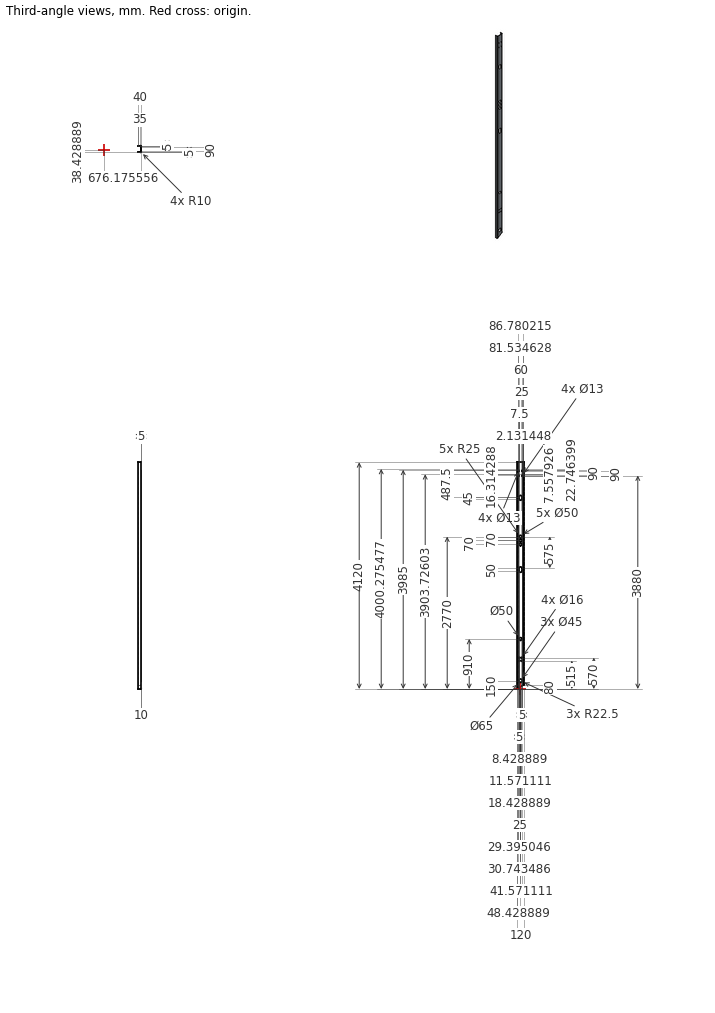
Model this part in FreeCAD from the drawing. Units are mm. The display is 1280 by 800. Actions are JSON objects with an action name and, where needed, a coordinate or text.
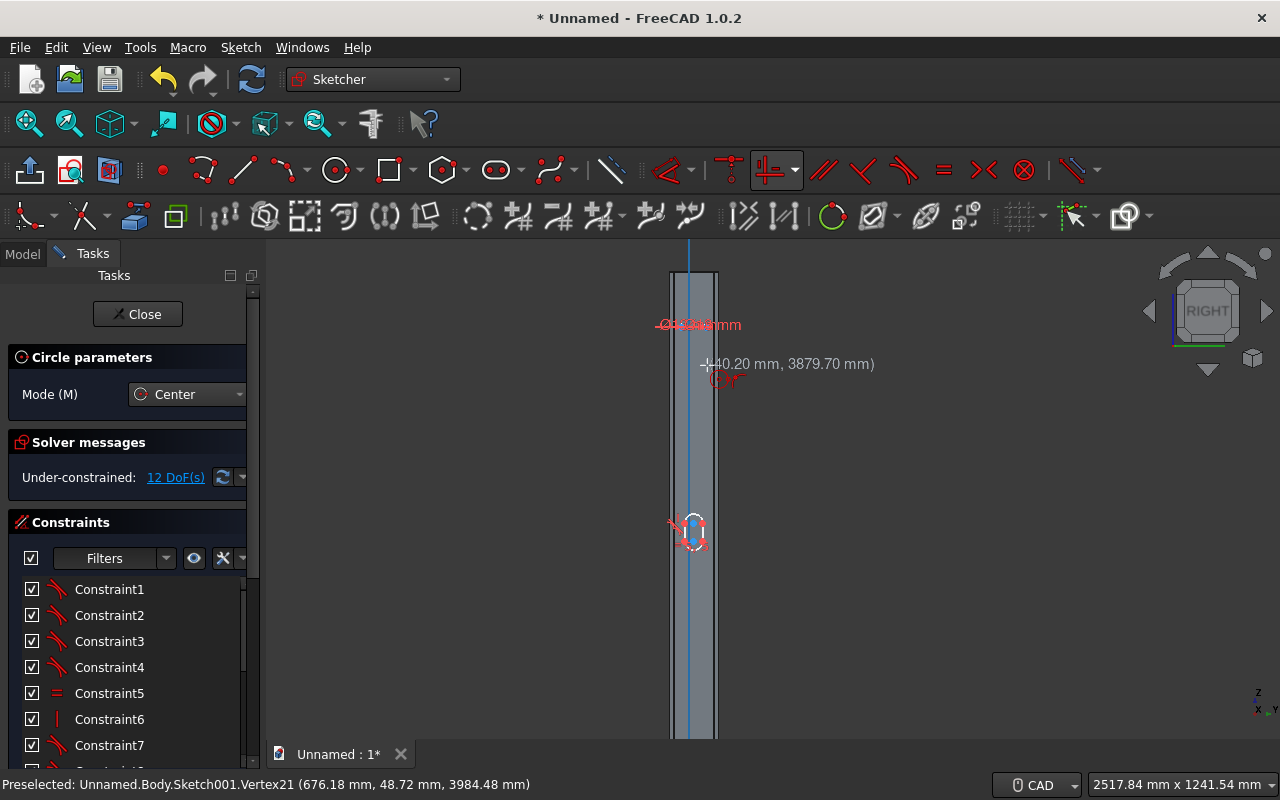
{"action": "left_click", "coordinate": [706, 363]}
{"action": "mouse_move", "coordinate": [708, 361]}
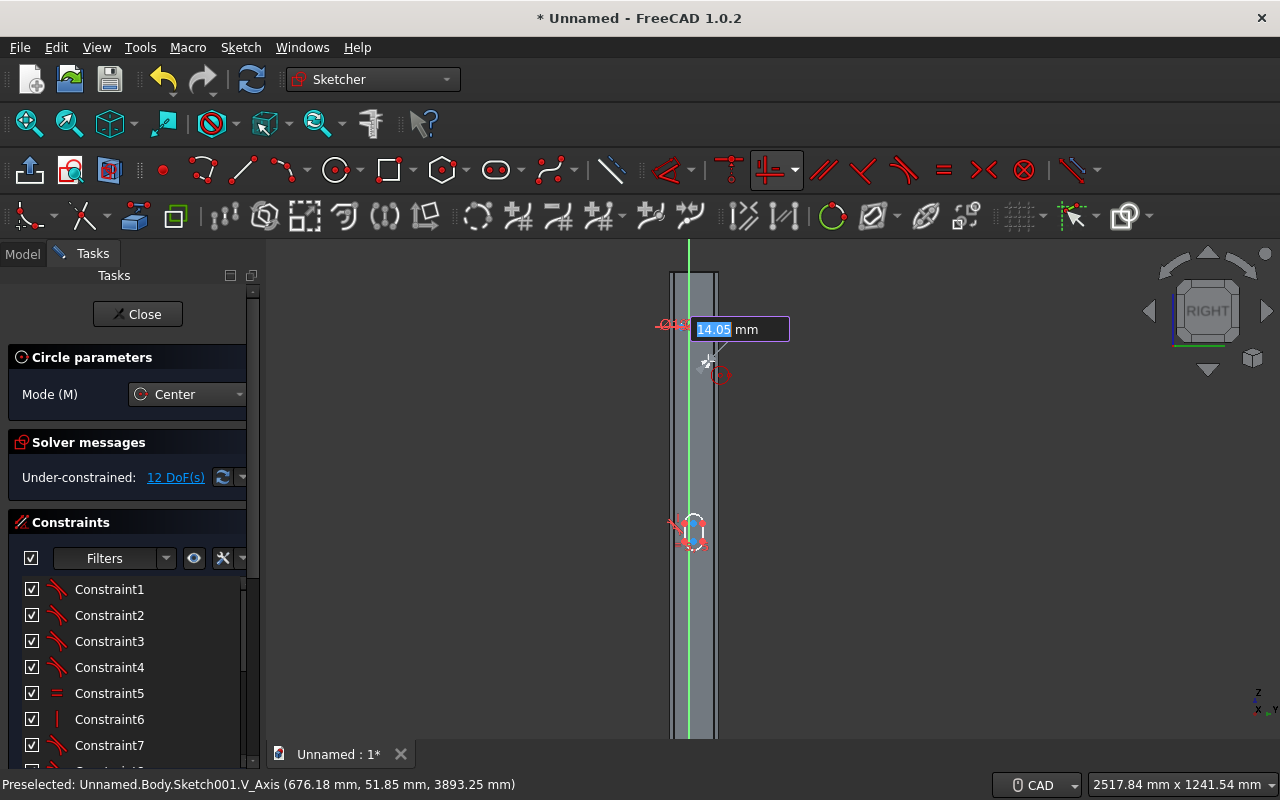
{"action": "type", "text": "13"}
{"action": "key", "text": "Return"}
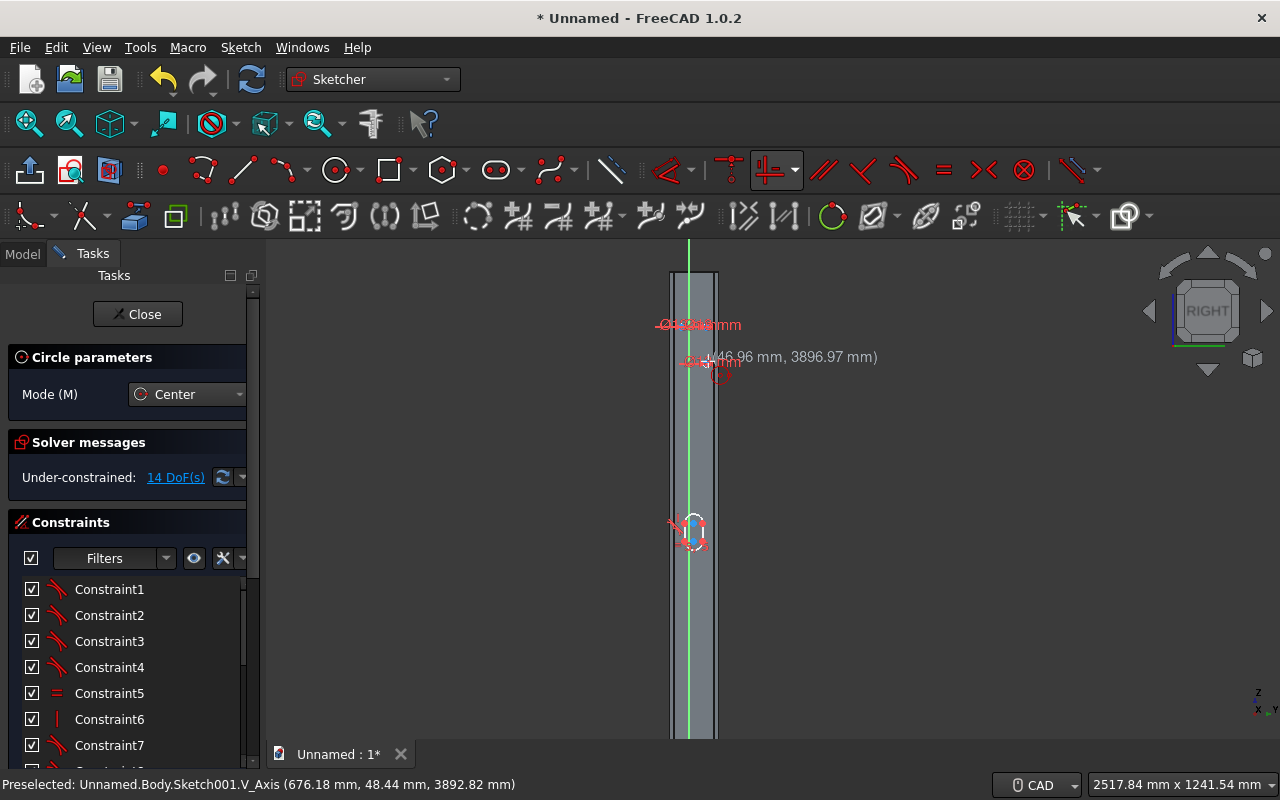
{"action": "scroll", "coordinate": [682, 363], "scroll_direction": "up", "scroll_amount": 11}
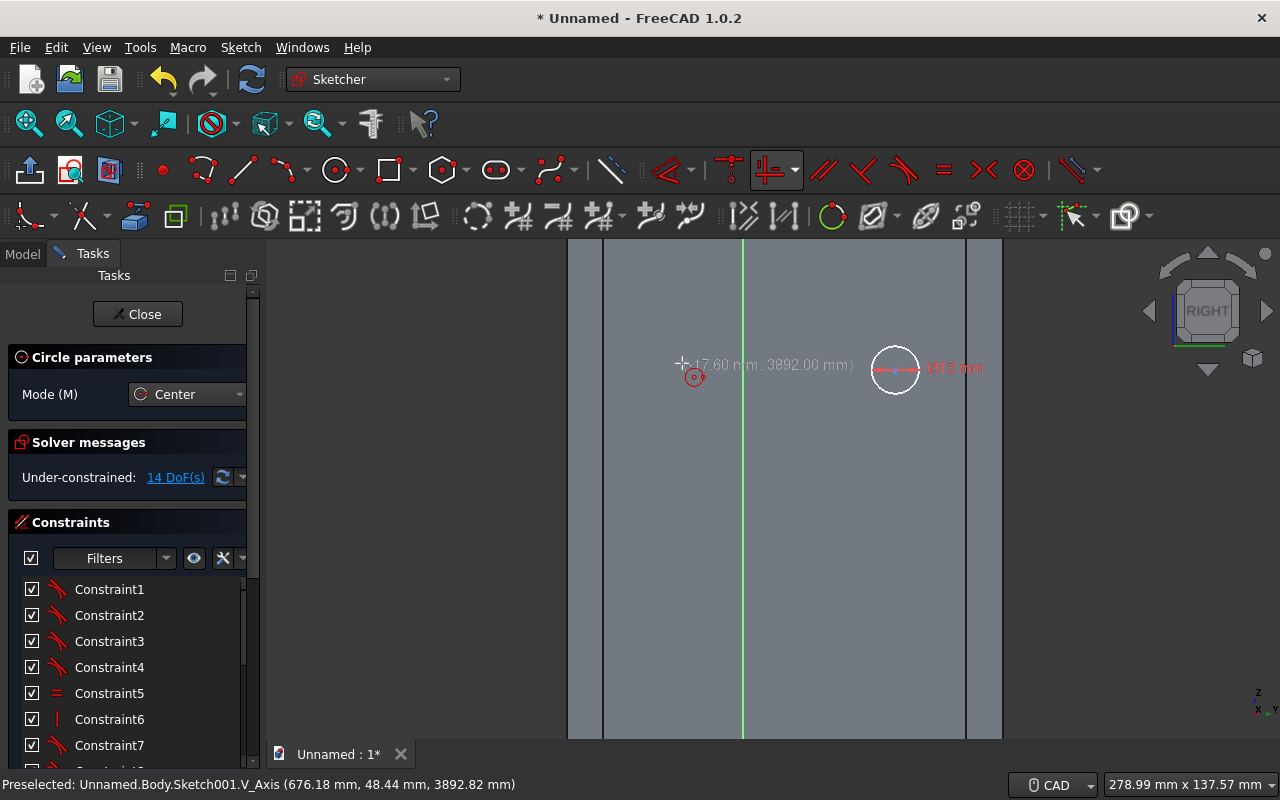
{"action": "scroll", "coordinate": [704, 489], "scroll_direction": "down", "scroll_amount": 15}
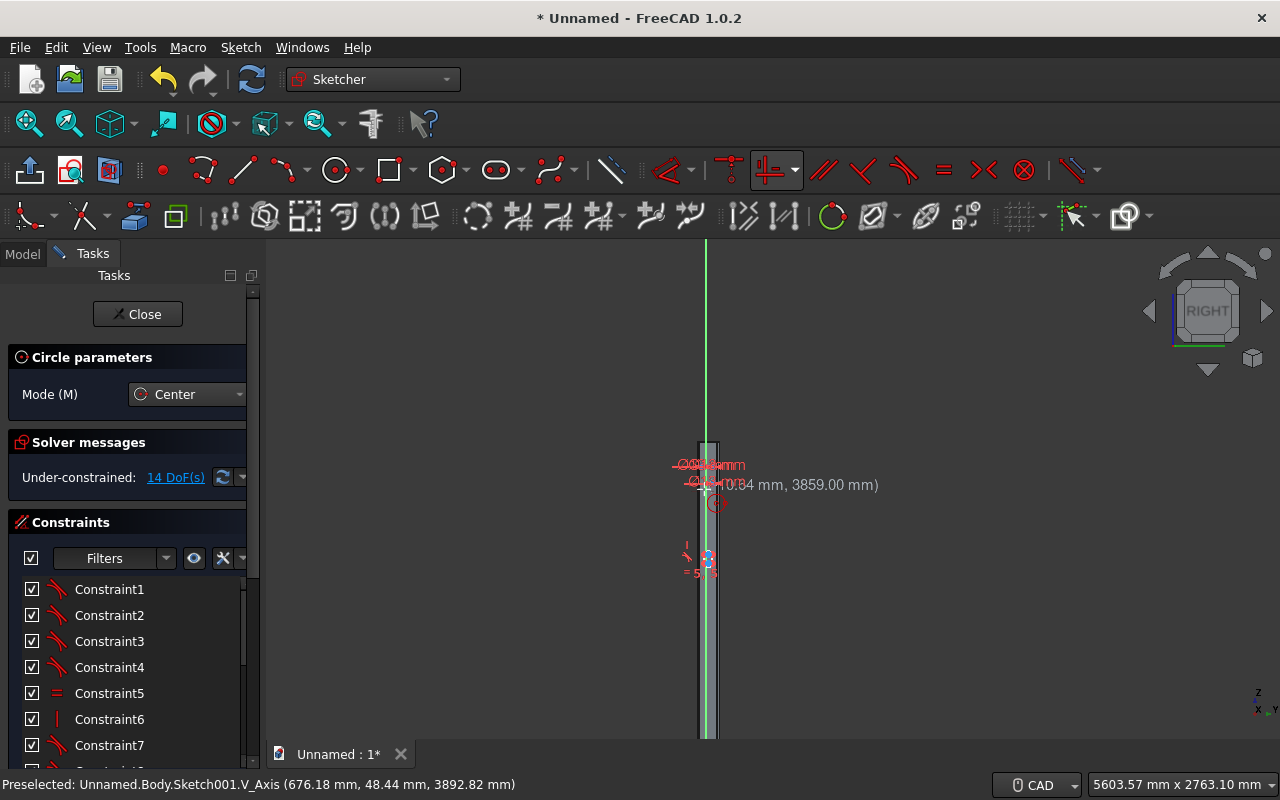
{"action": "scroll", "coordinate": [701, 267], "scroll_direction": "down", "scroll_amount": 4}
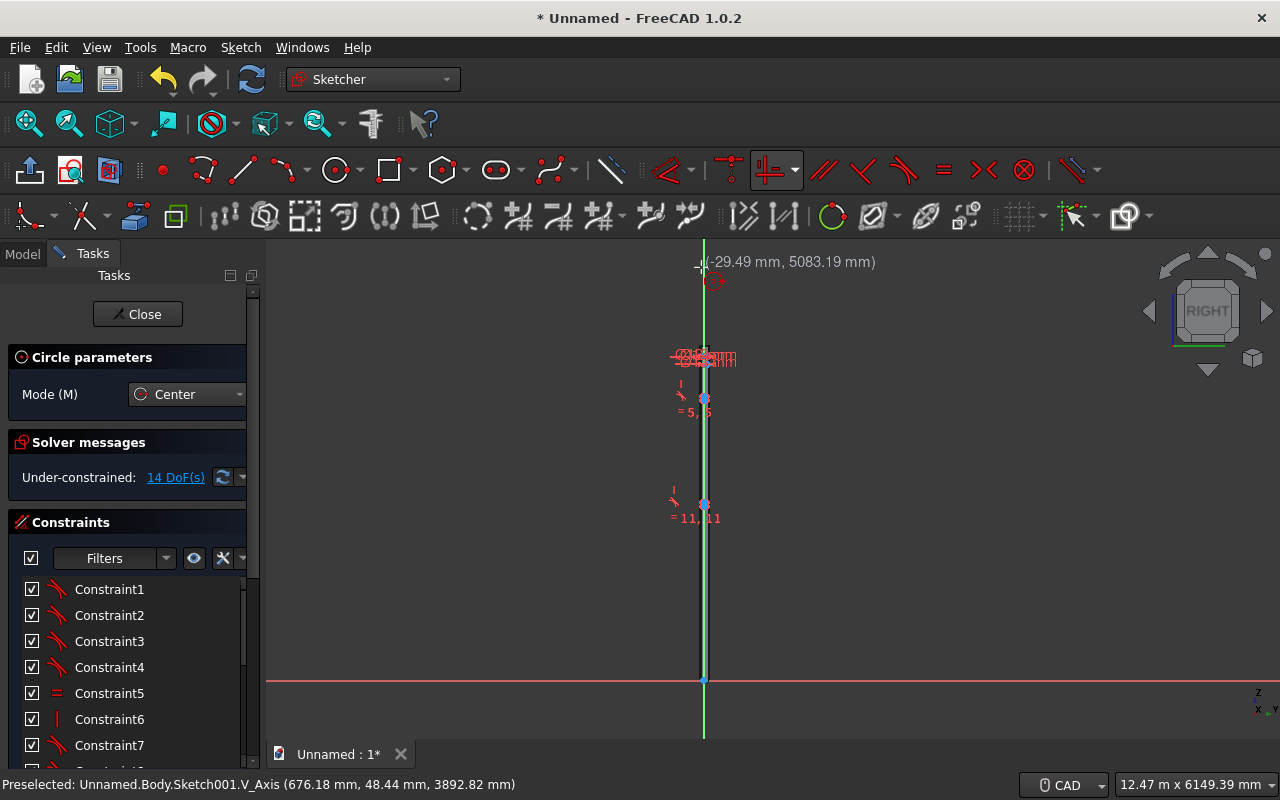
{"action": "scroll", "coordinate": [702, 364], "scroll_direction": "up", "scroll_amount": 12}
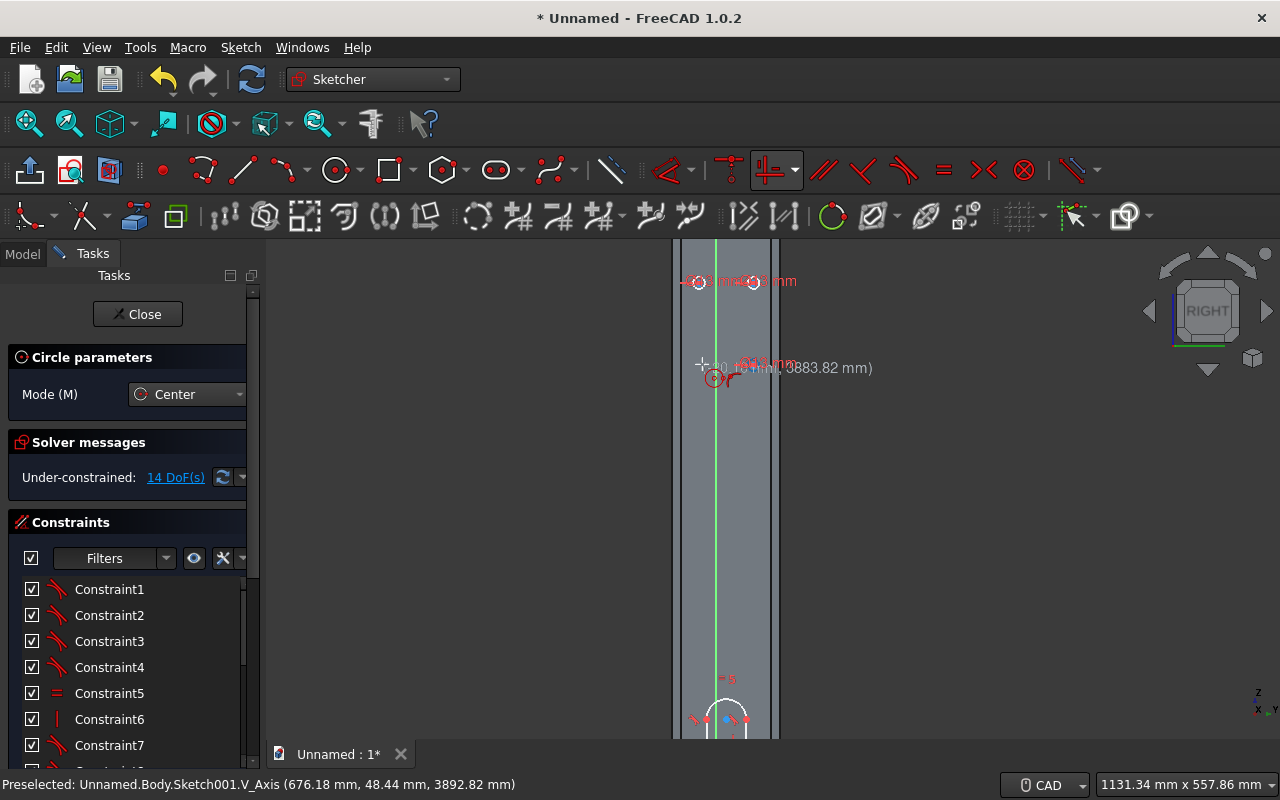
{"action": "left_click", "coordinate": [699, 362]}
{"action": "mouse_move", "coordinate": [695, 358]}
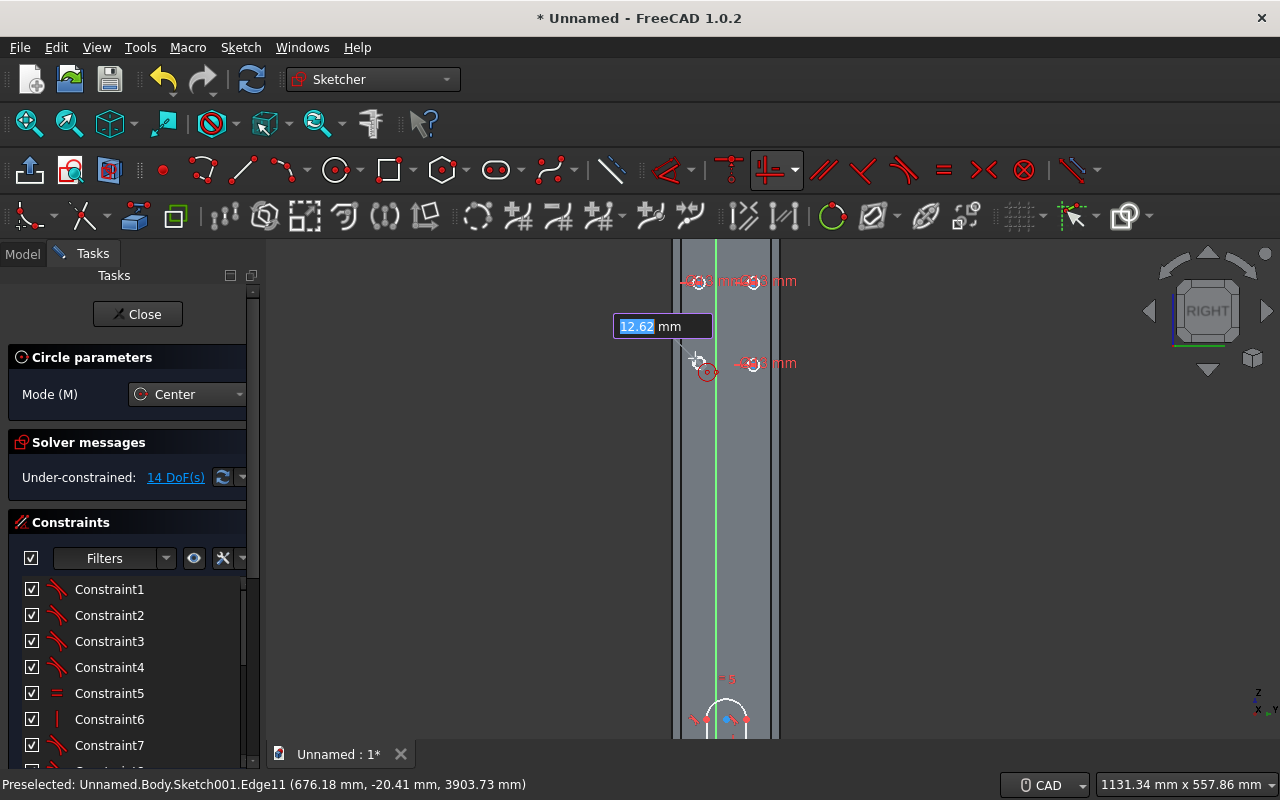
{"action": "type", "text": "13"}
{"action": "key", "text": "Return"}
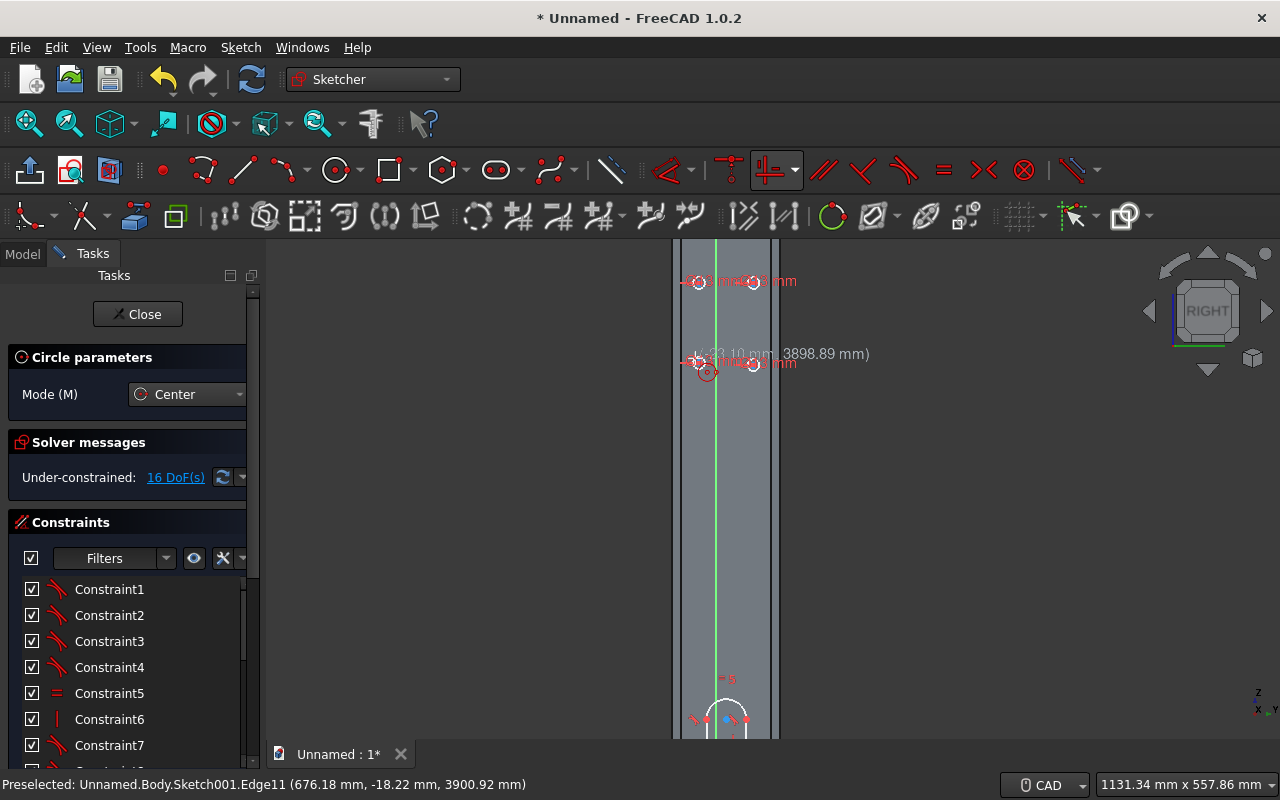
{"action": "scroll", "coordinate": [702, 332], "scroll_direction": "down", "scroll_amount": 12}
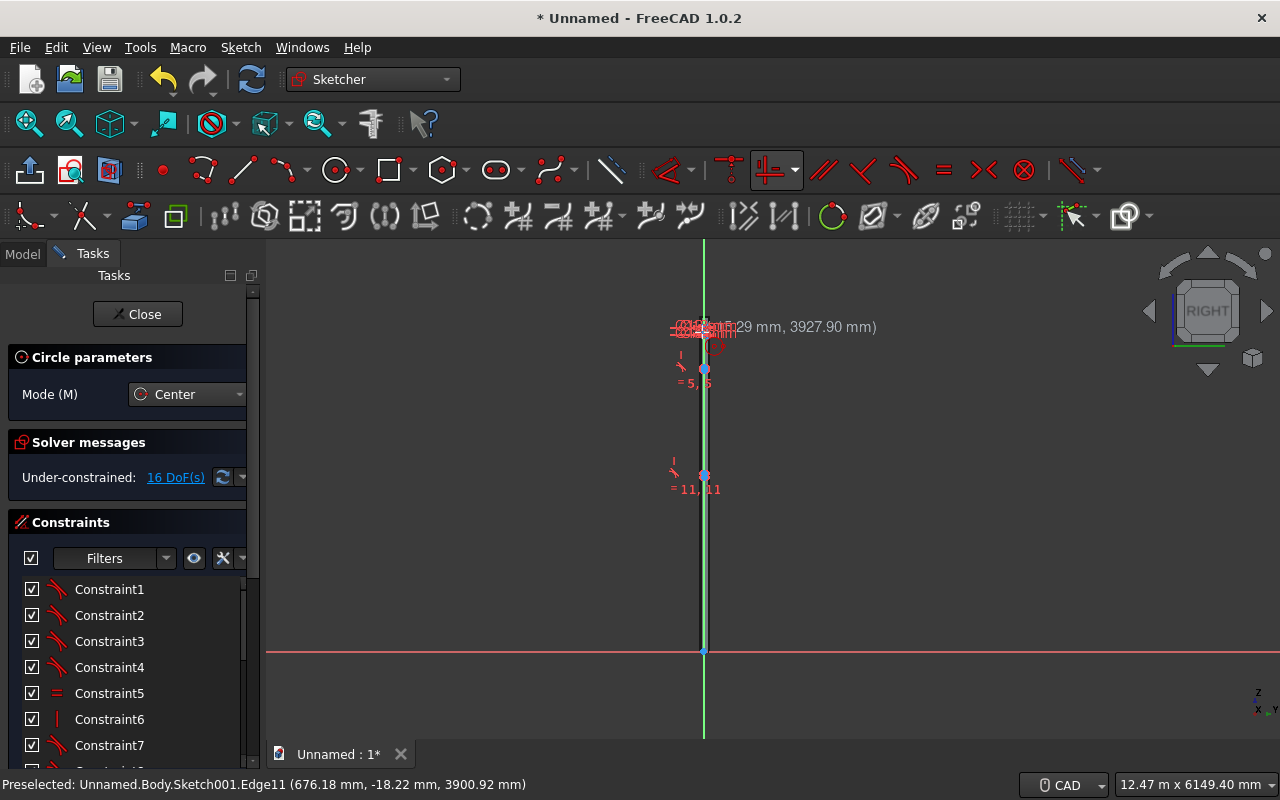
{"action": "scroll", "coordinate": [705, 426], "scroll_direction": "up", "scroll_amount": 15}